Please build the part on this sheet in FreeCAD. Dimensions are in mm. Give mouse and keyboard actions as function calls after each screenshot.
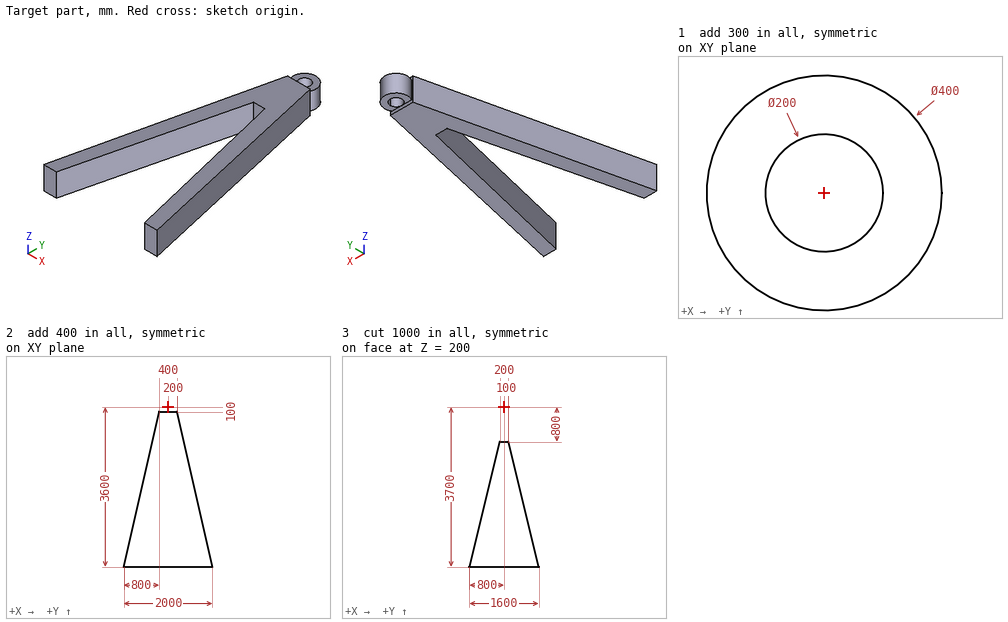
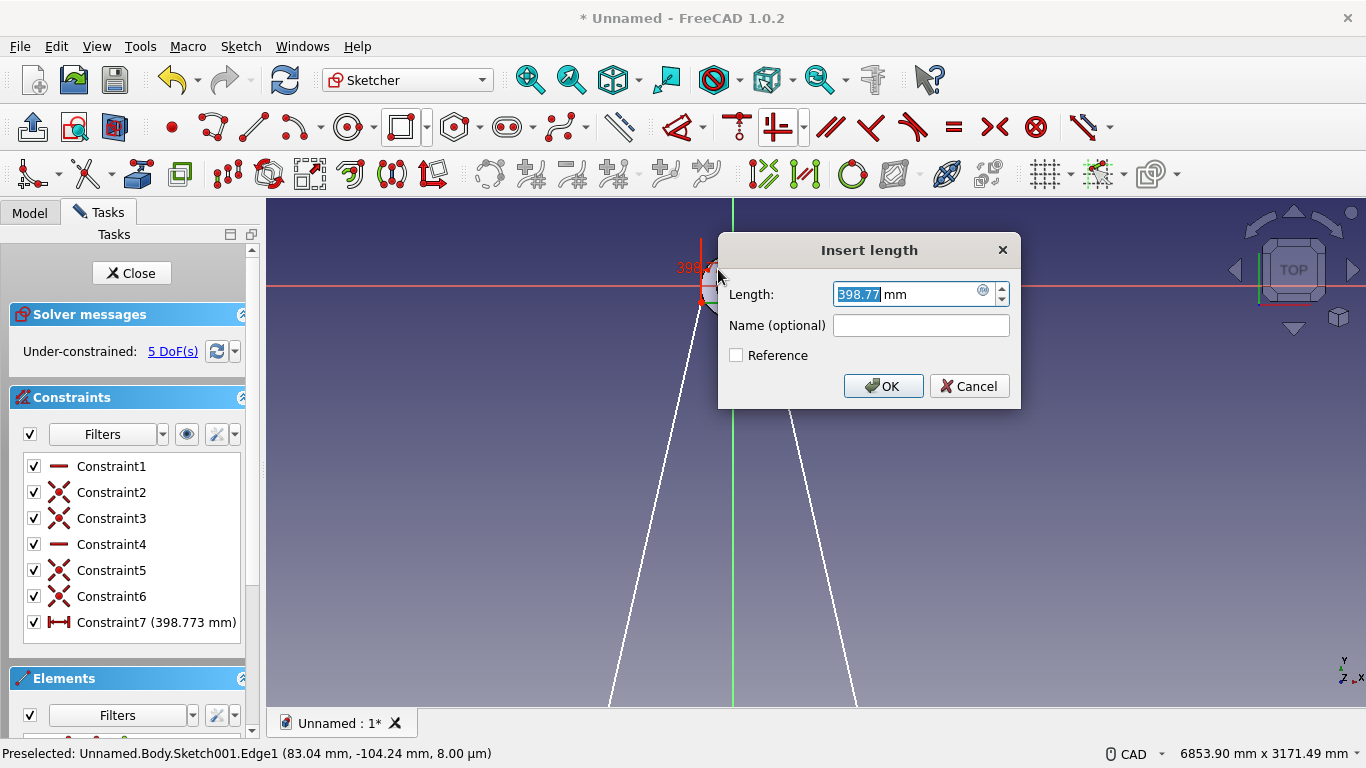
text(400)
key(Return)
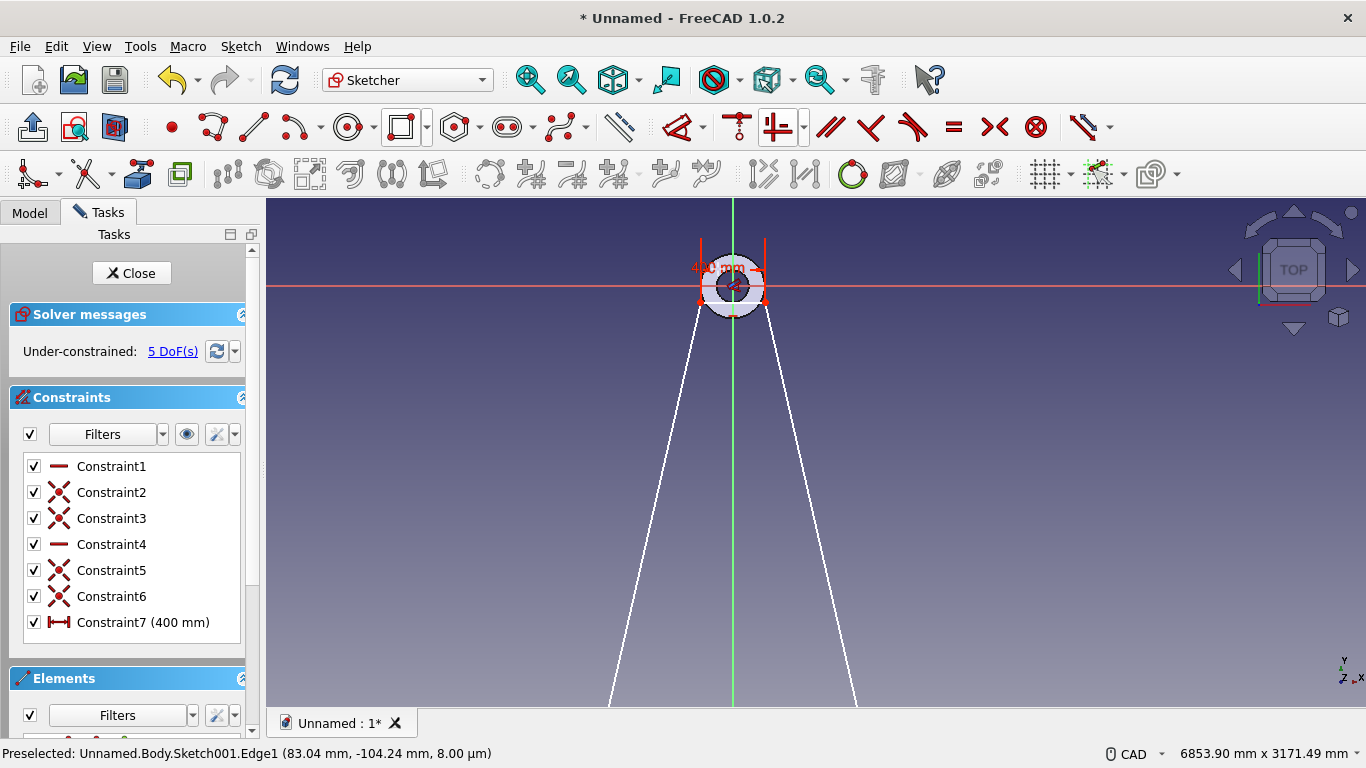
scroll(766, 303, down, 3)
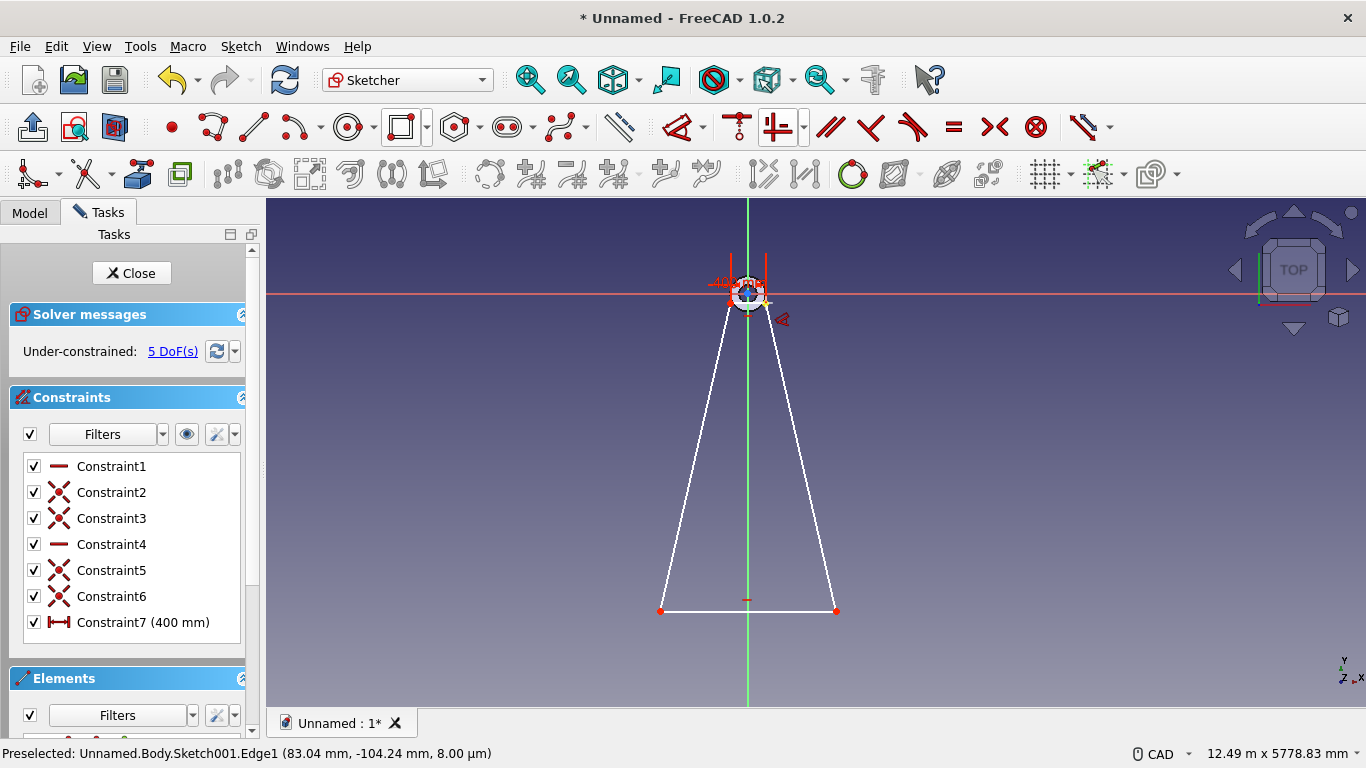
click(713, 612)
click(708, 646)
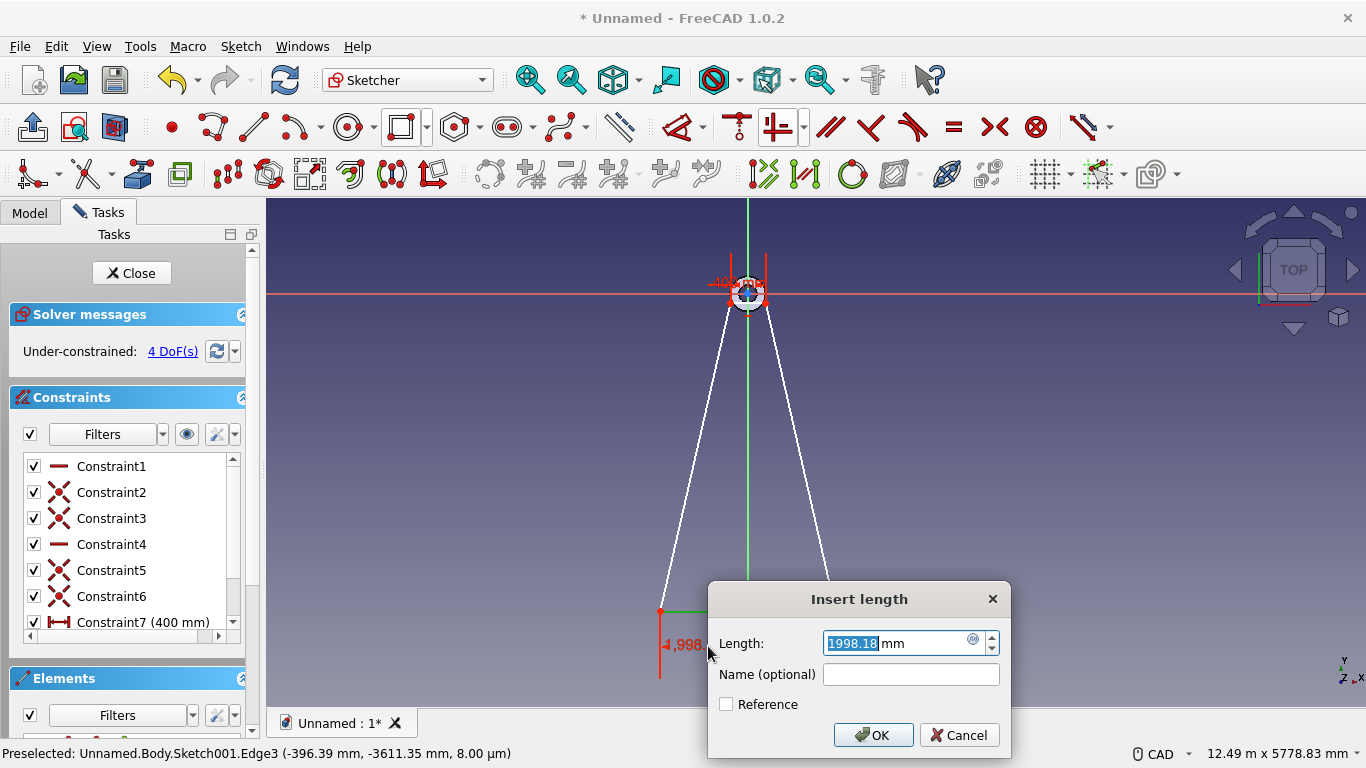
text(2000)
key(Return)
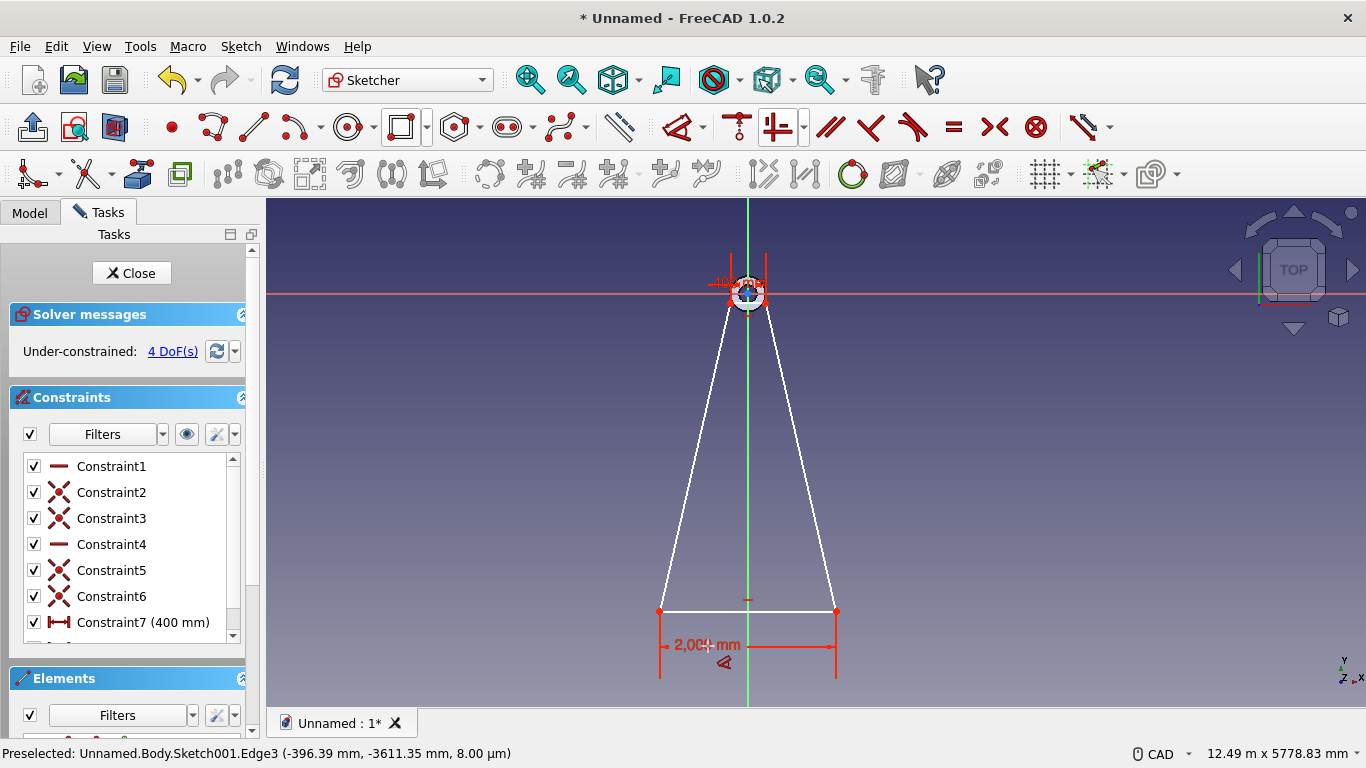
scroll(766, 303, up, 5)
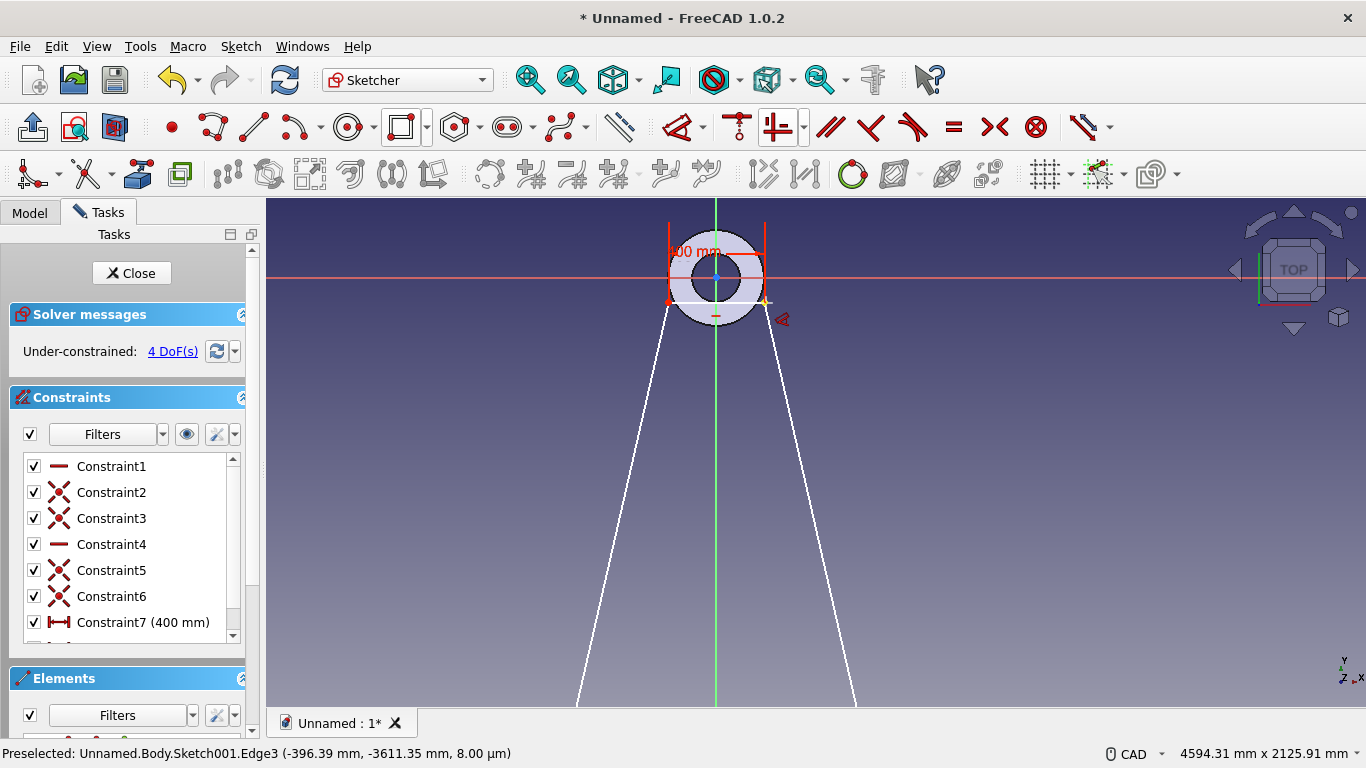
click(765, 303)
click(740, 337)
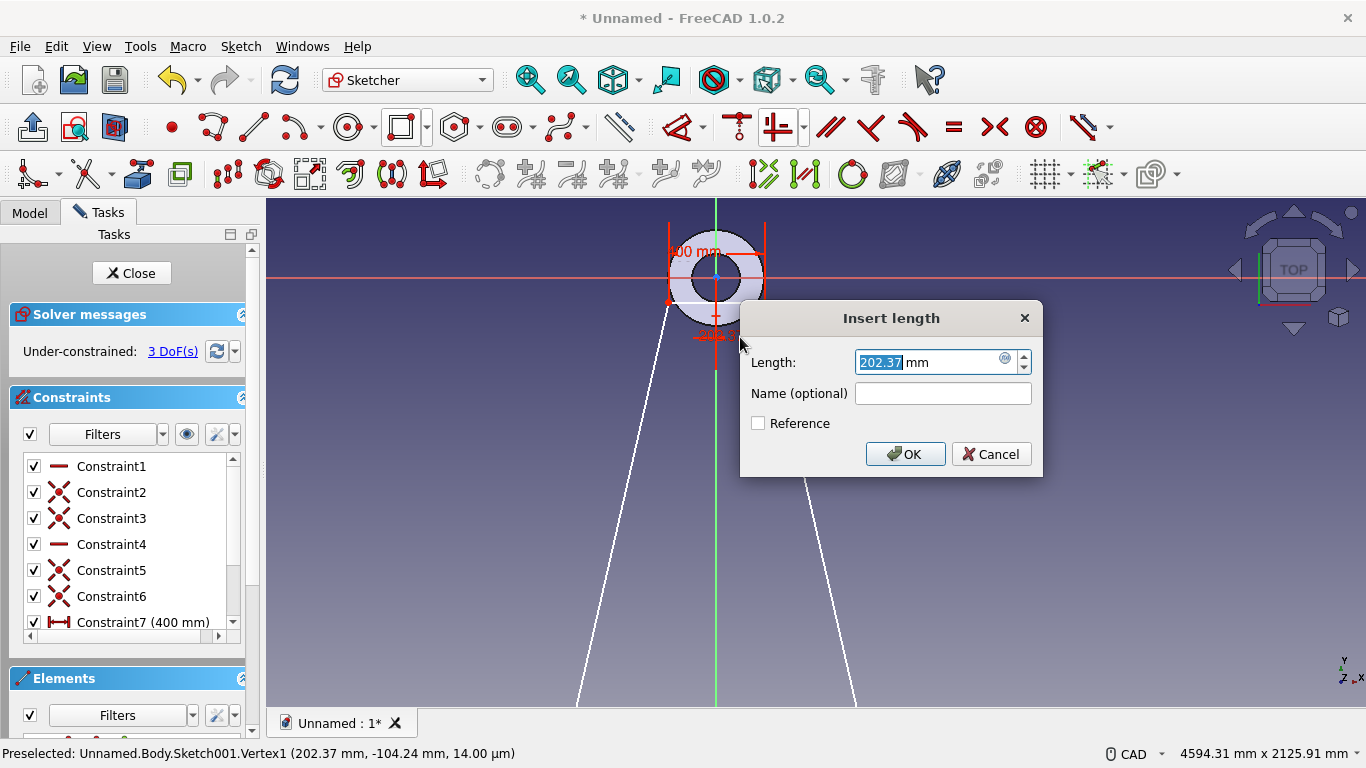
text(200)
key(Return)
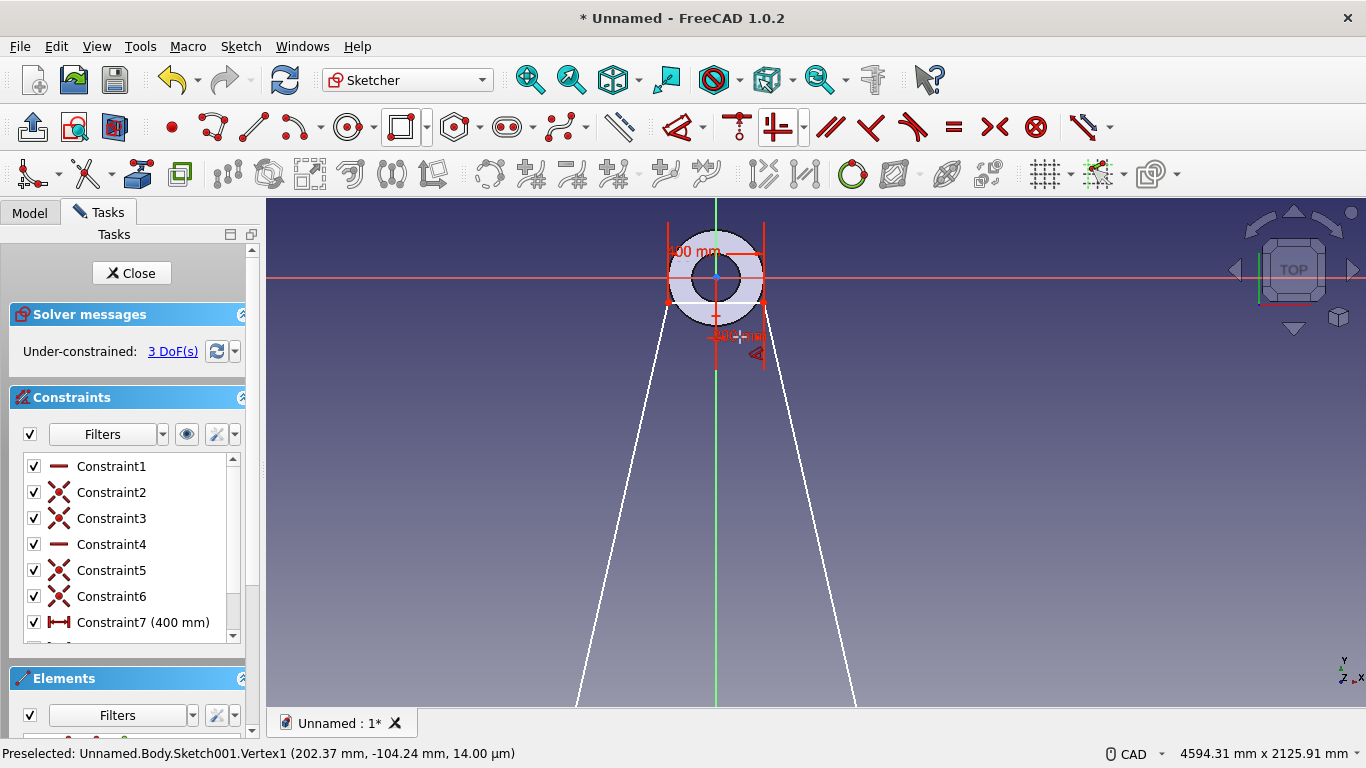
scroll(764, 303, up, 3)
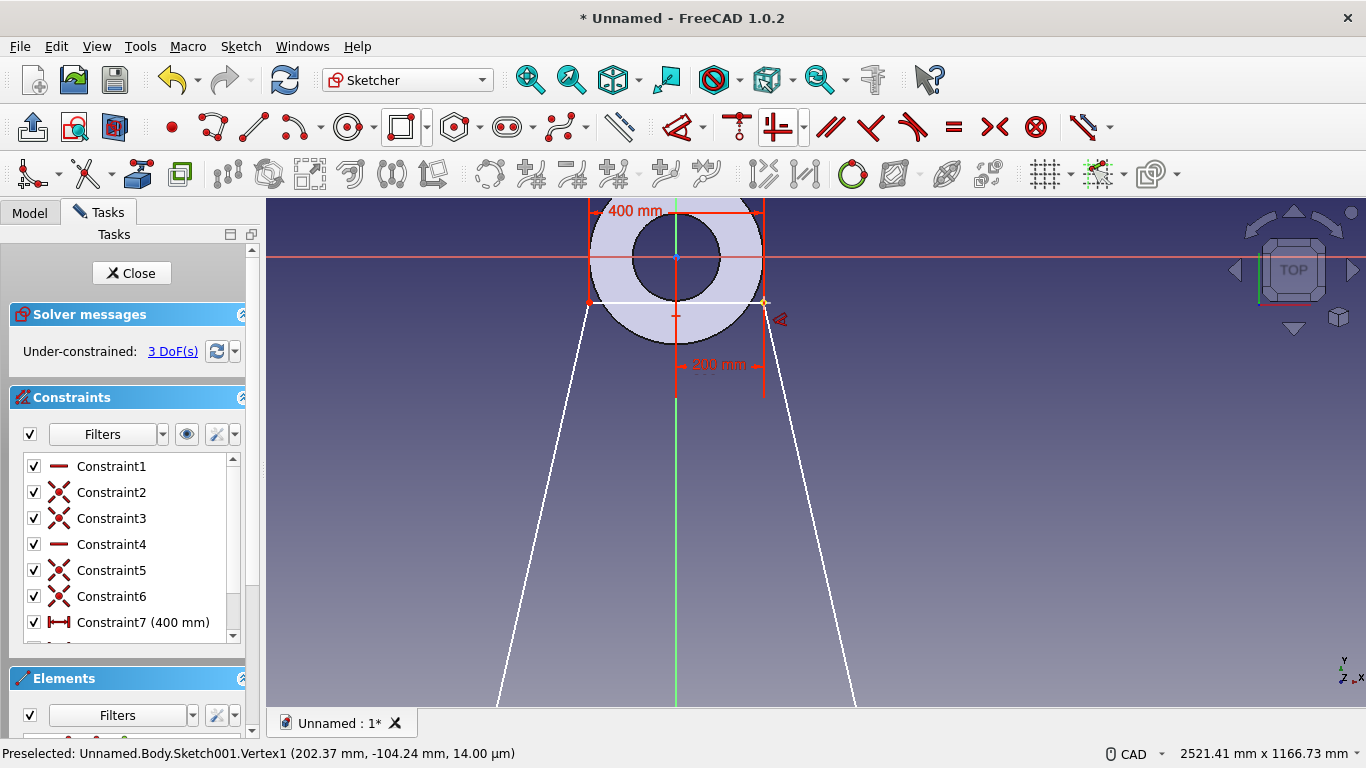
click(764, 303)
click(798, 280)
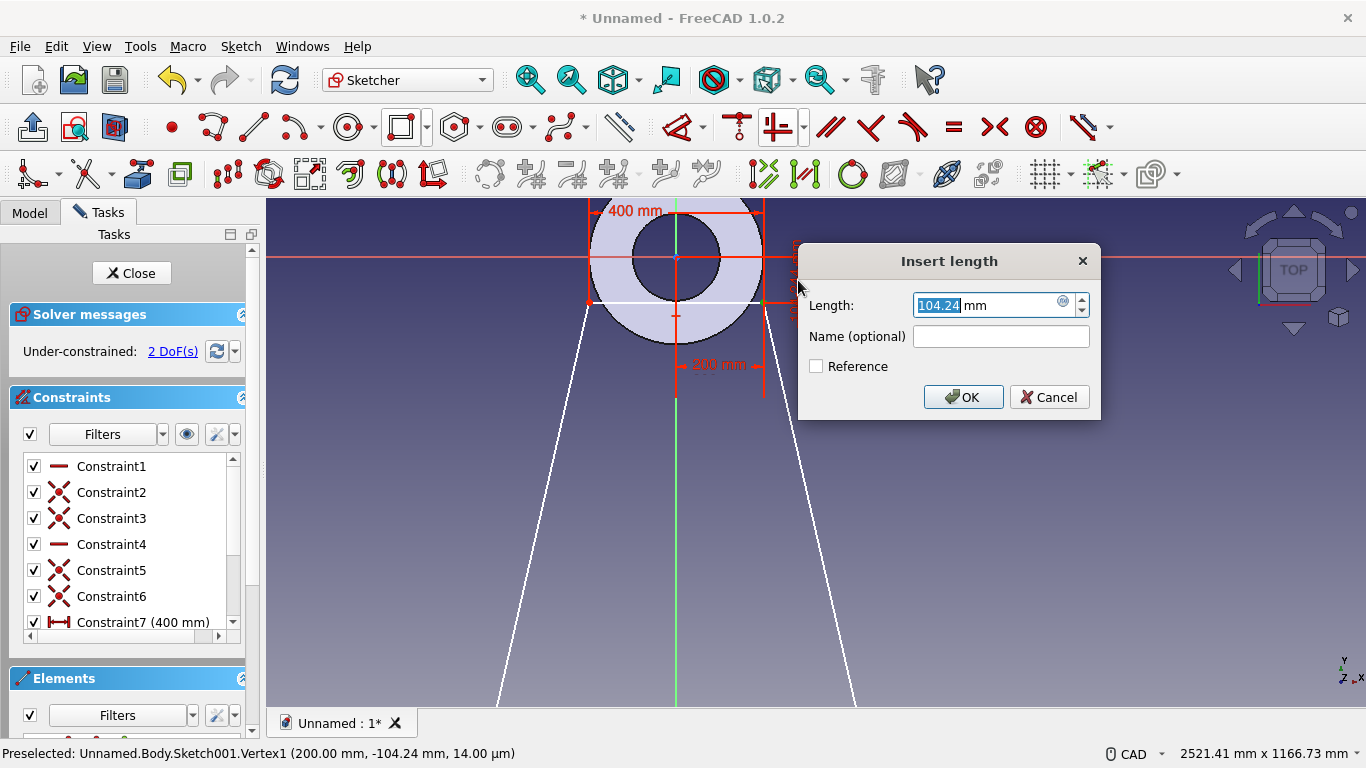
text(100)
key(Return)